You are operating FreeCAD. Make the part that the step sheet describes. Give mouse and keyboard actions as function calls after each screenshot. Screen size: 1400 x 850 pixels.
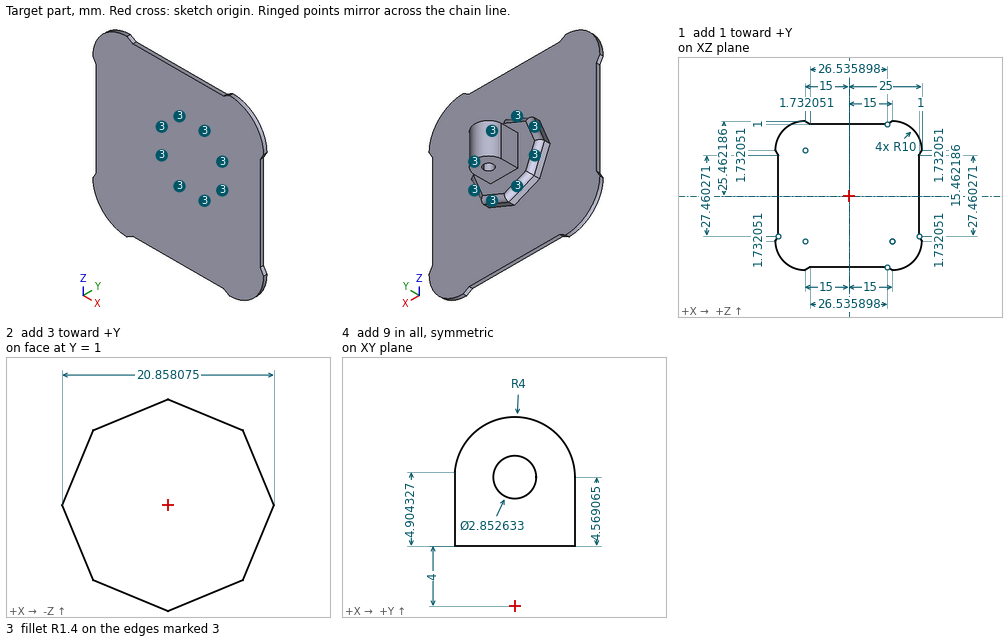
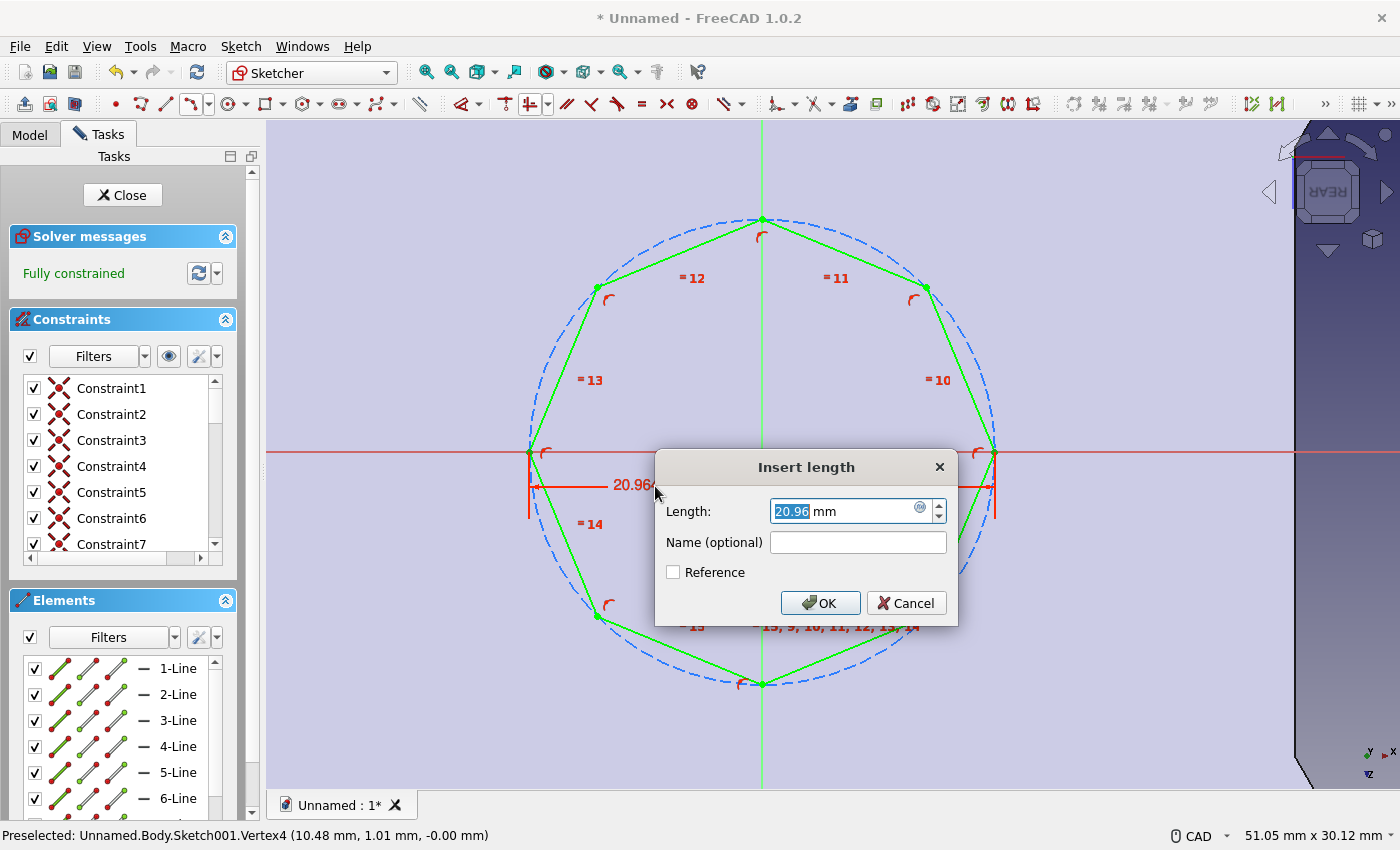
text(20.858075)
key(Return)
key(Escape)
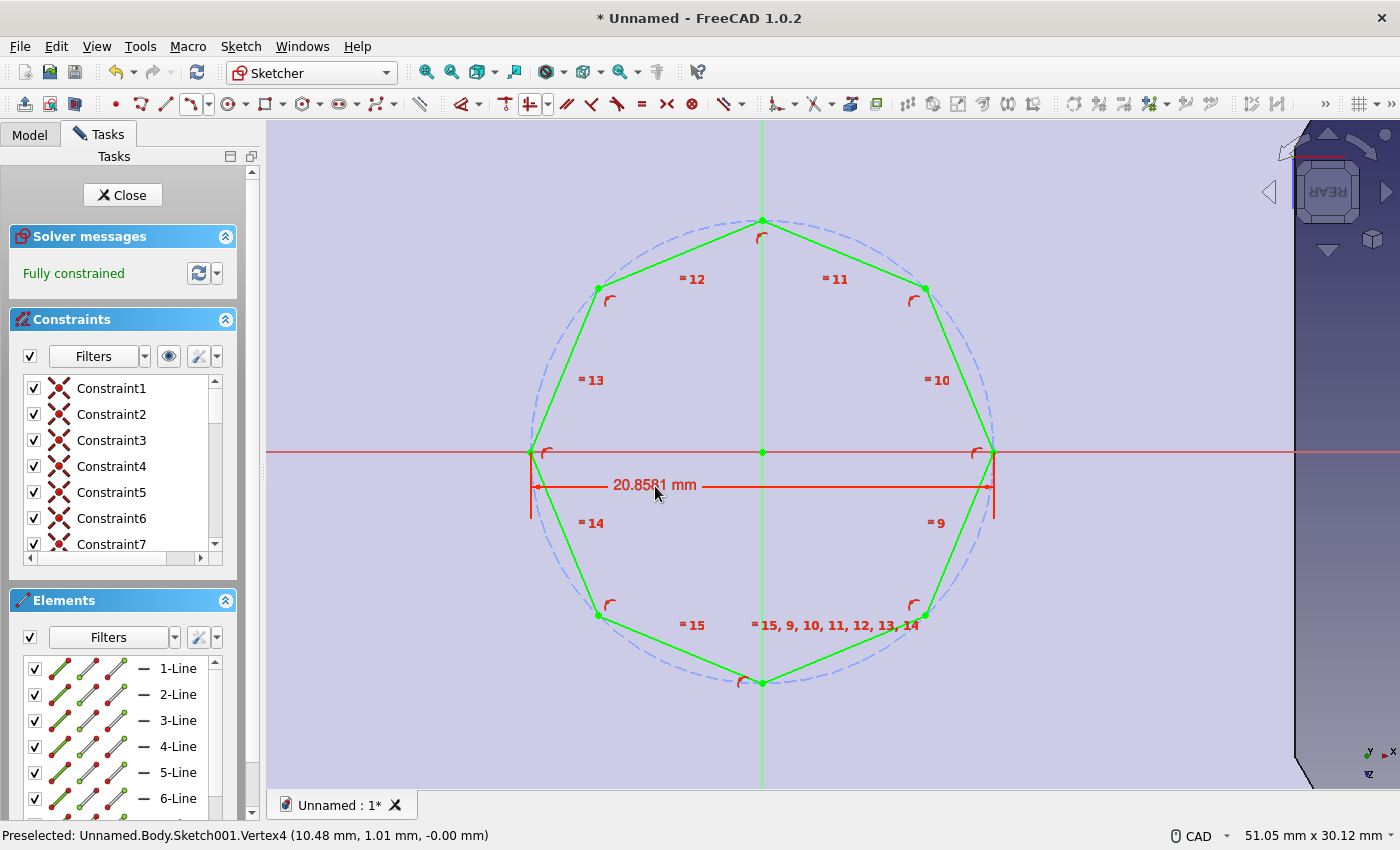
click(123, 195)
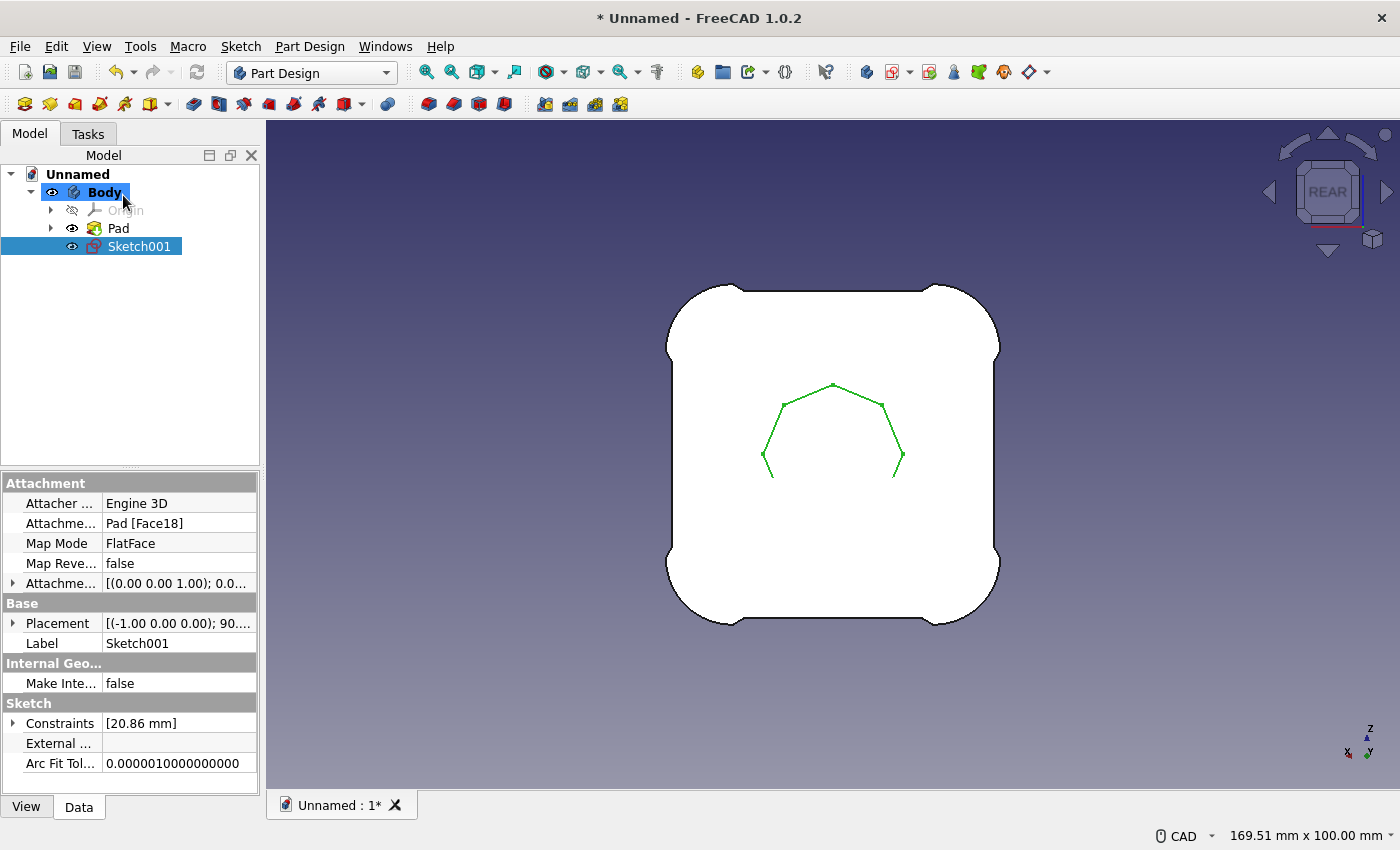
click(25, 104)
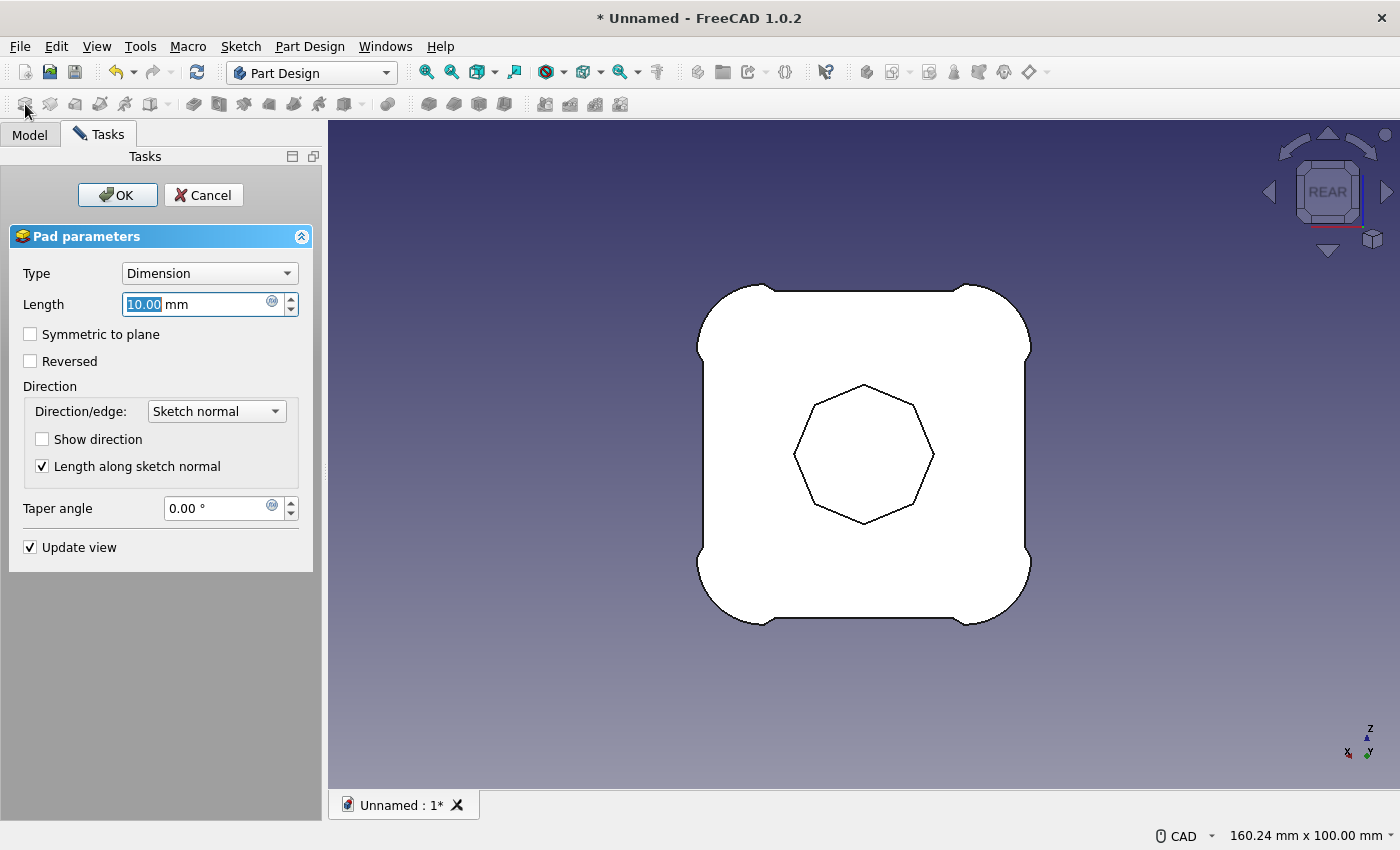
text(3)
key(Tab)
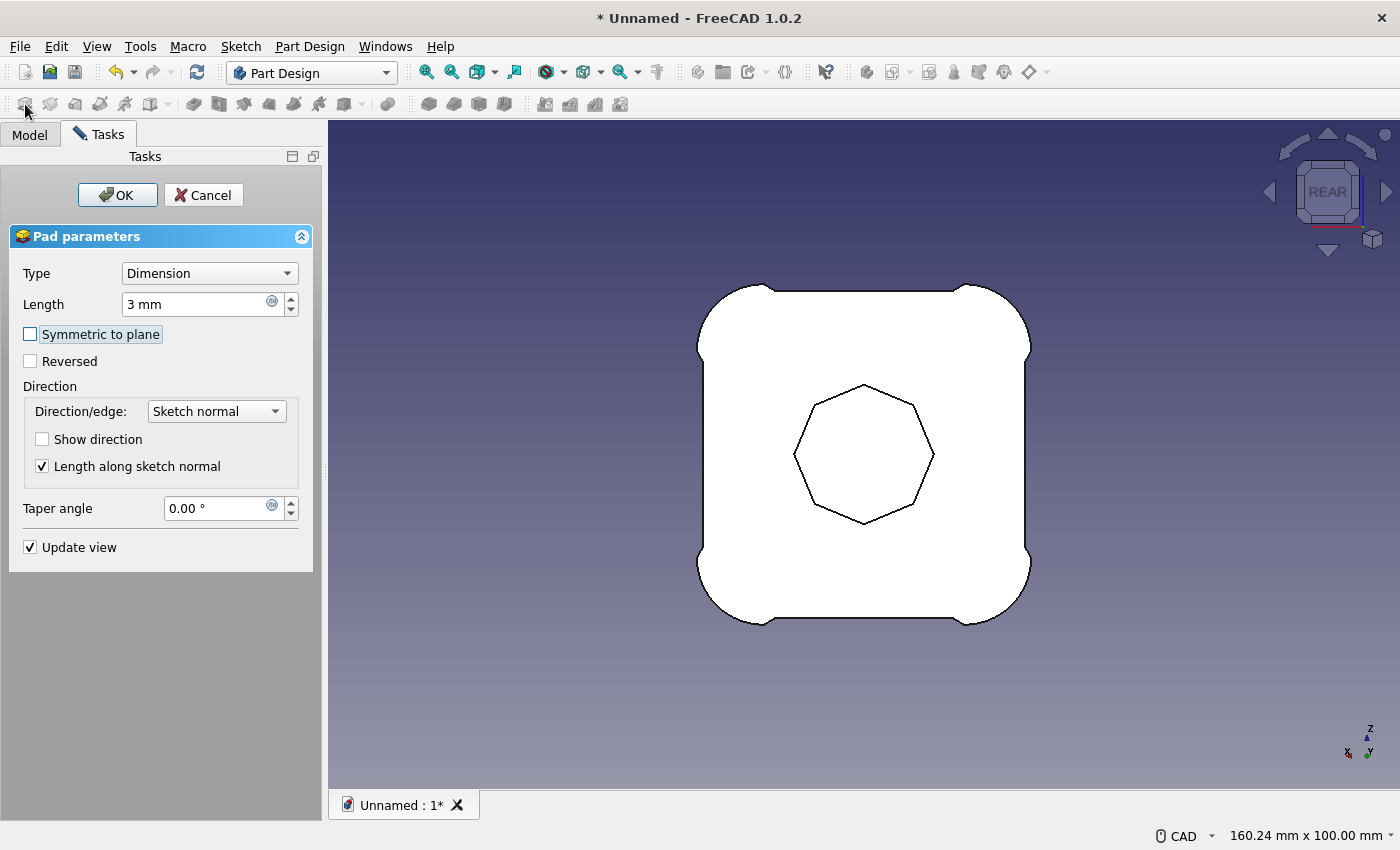
click(118, 195)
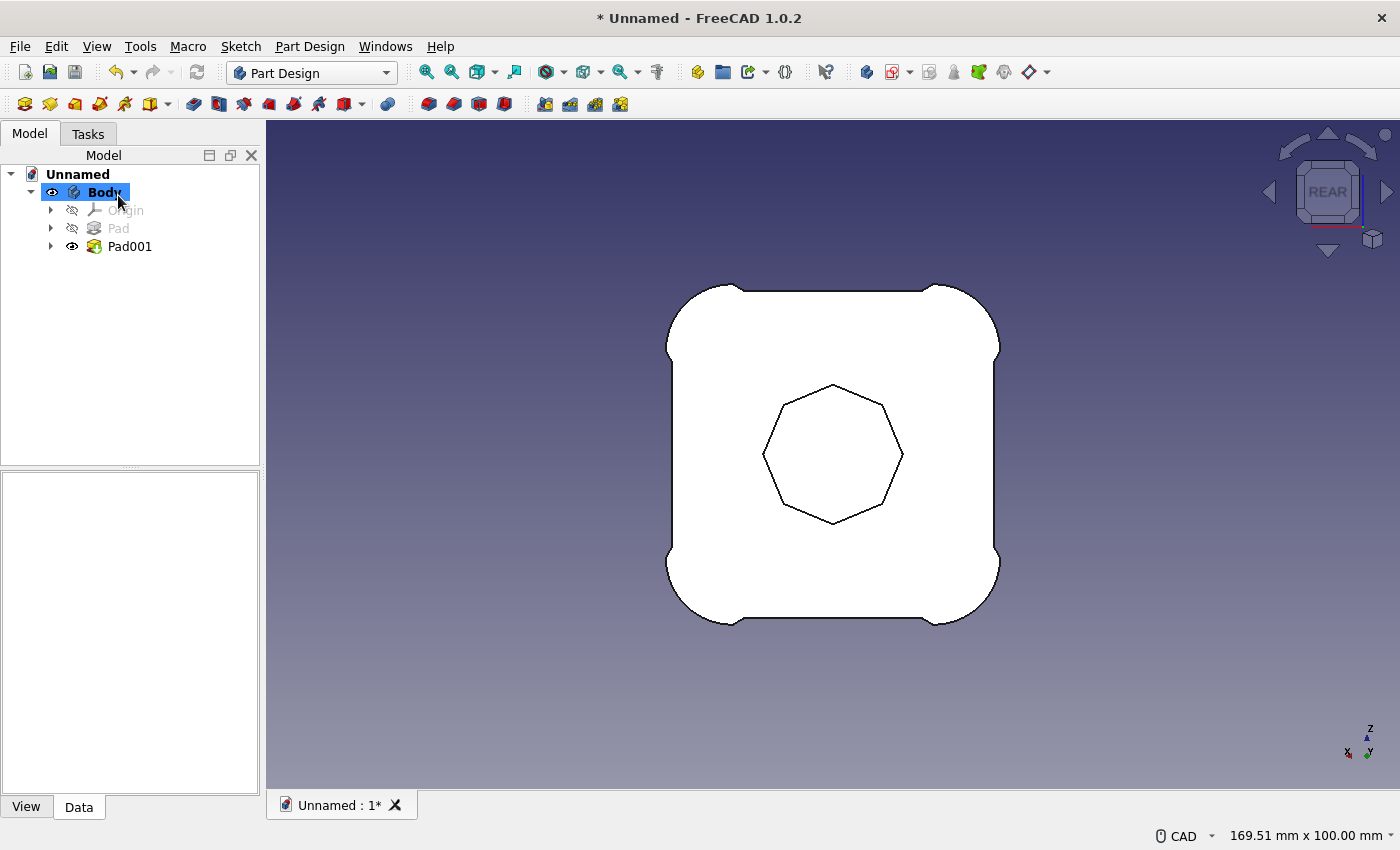
click(833, 453)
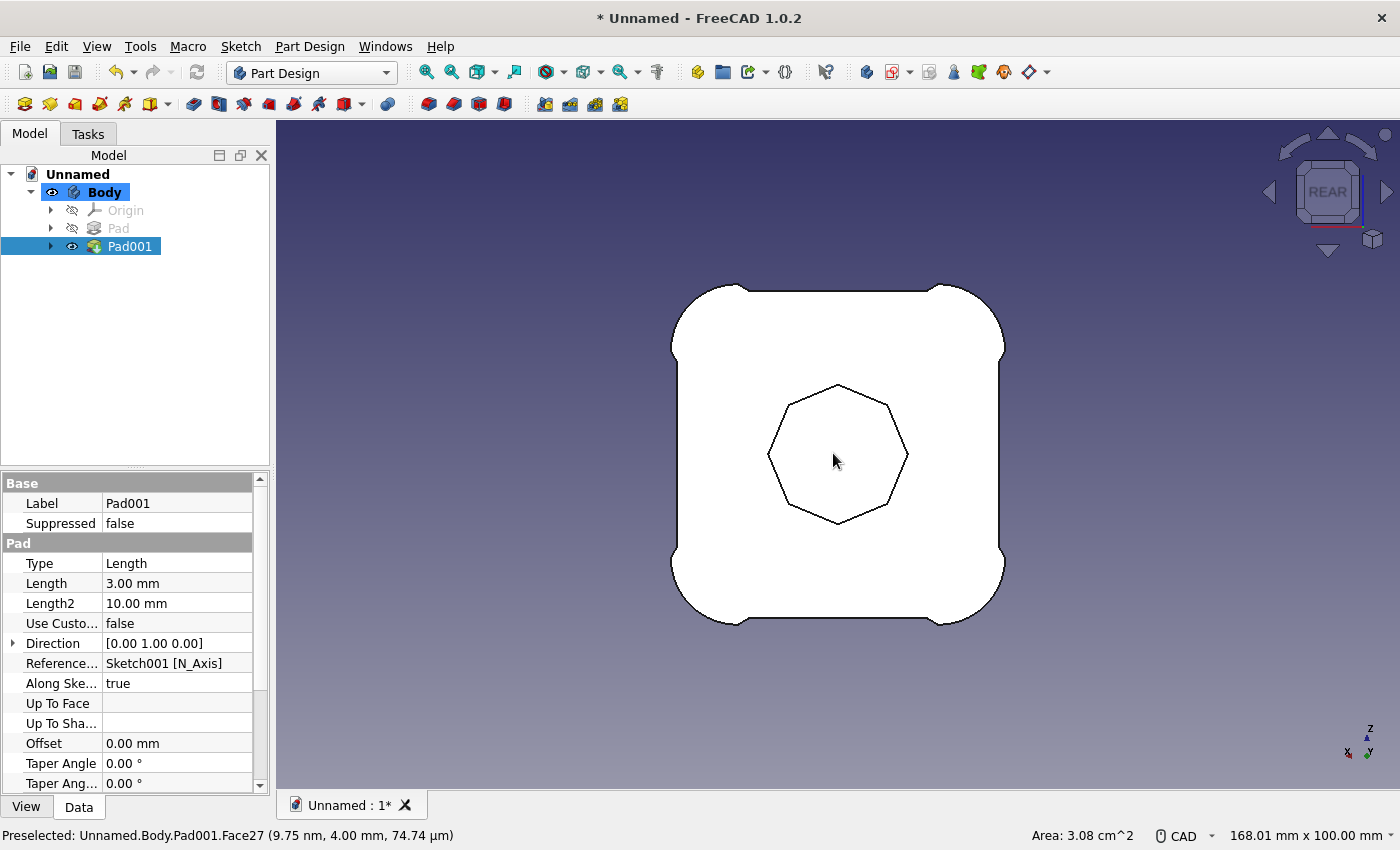
click(429, 104)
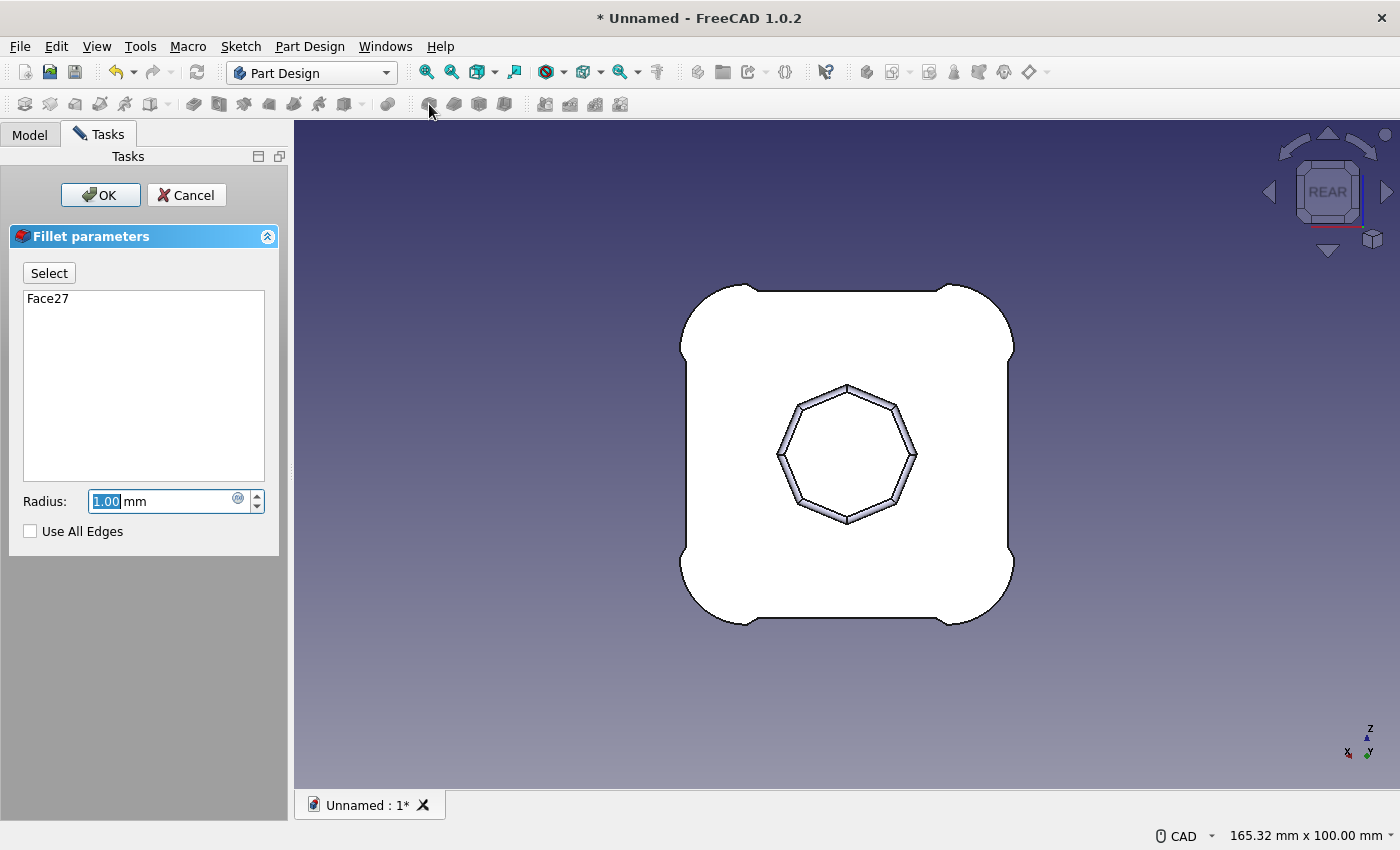
text(1.4)
key(Tab)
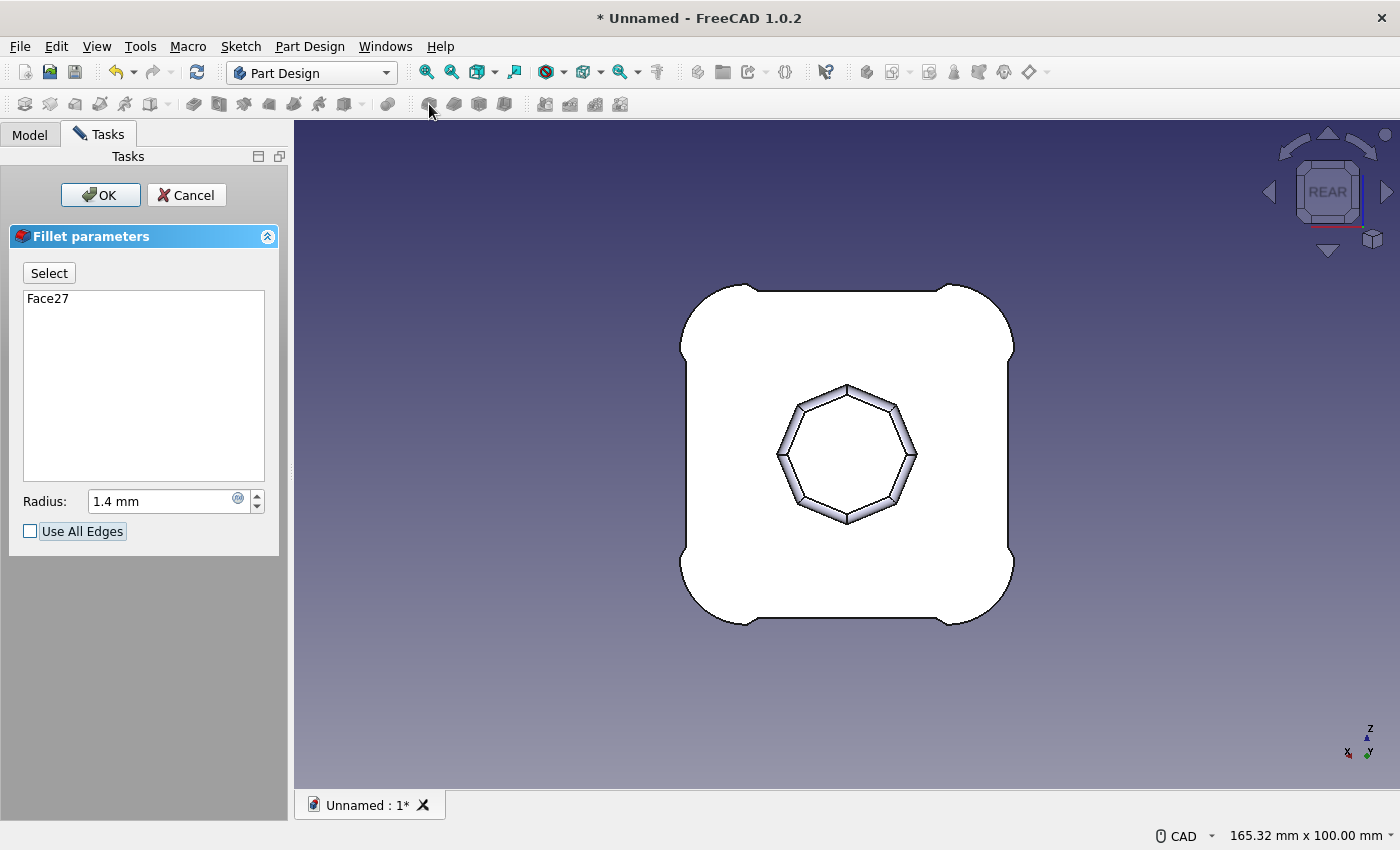
click(101, 195)